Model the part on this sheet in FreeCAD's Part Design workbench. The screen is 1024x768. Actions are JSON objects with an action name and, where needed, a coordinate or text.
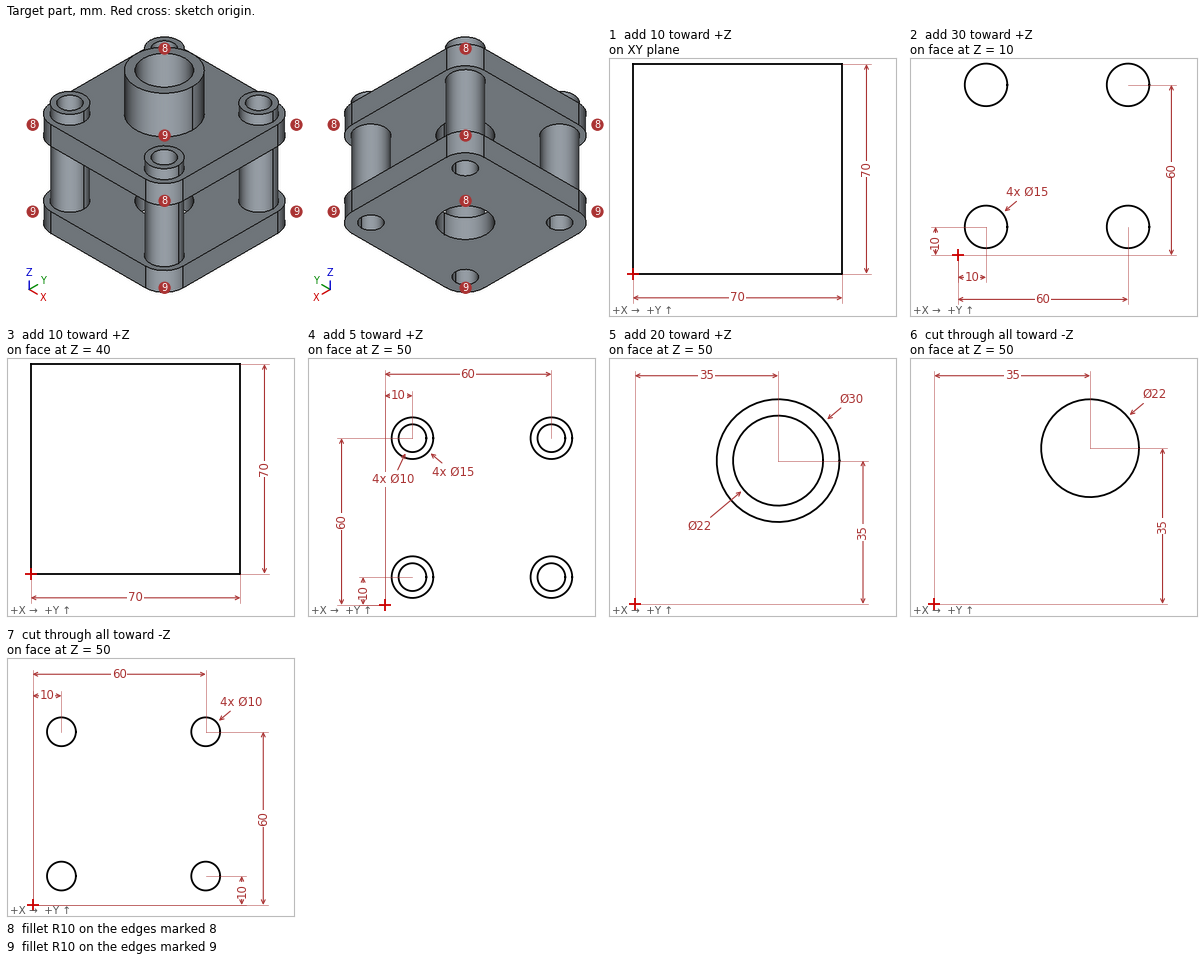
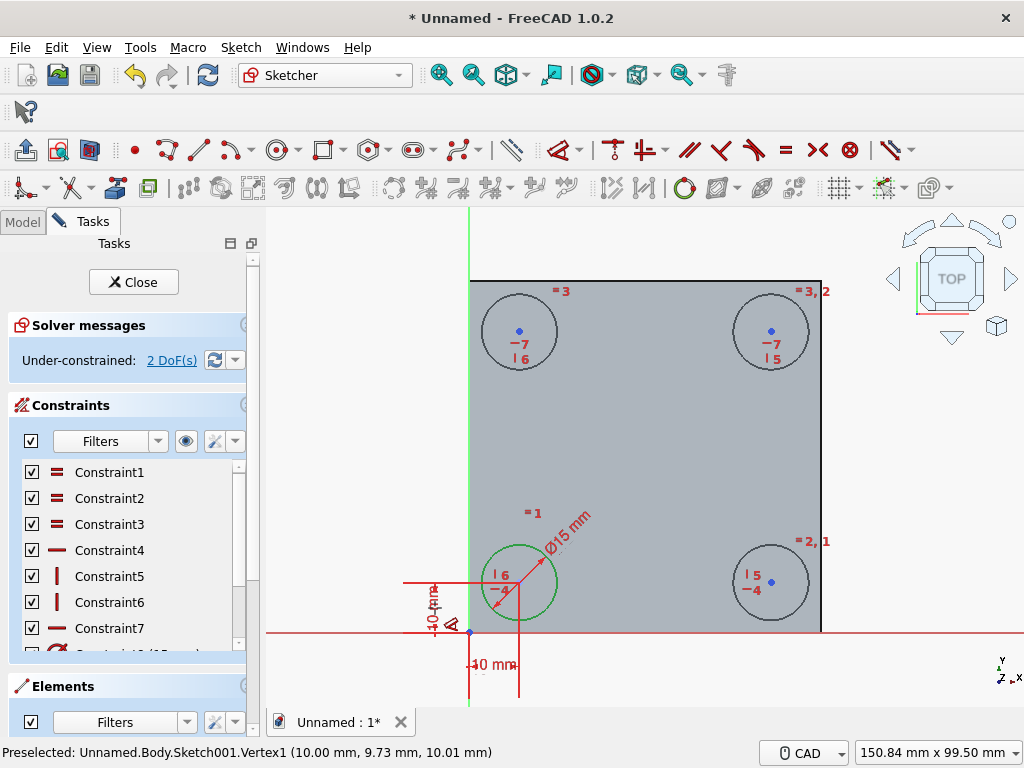
{"action": "left_click", "coordinate": [771, 583]}
{"action": "left_click", "coordinate": [620, 667]}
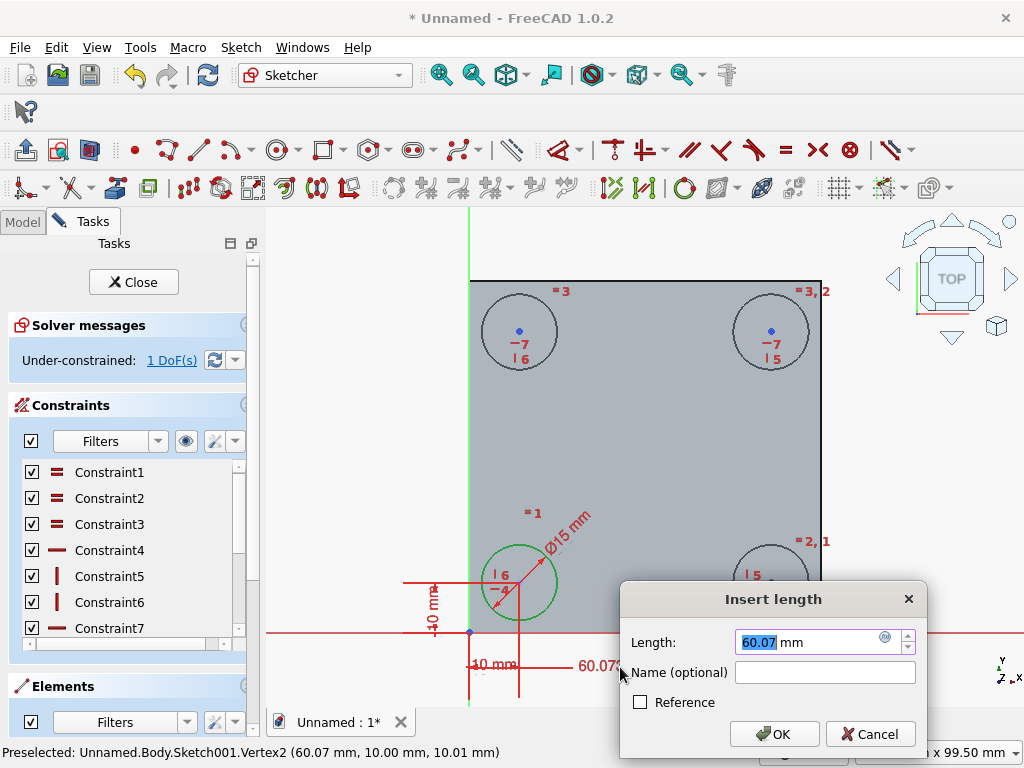
{"action": "type", "text": "60"}
{"action": "key", "text": "Return"}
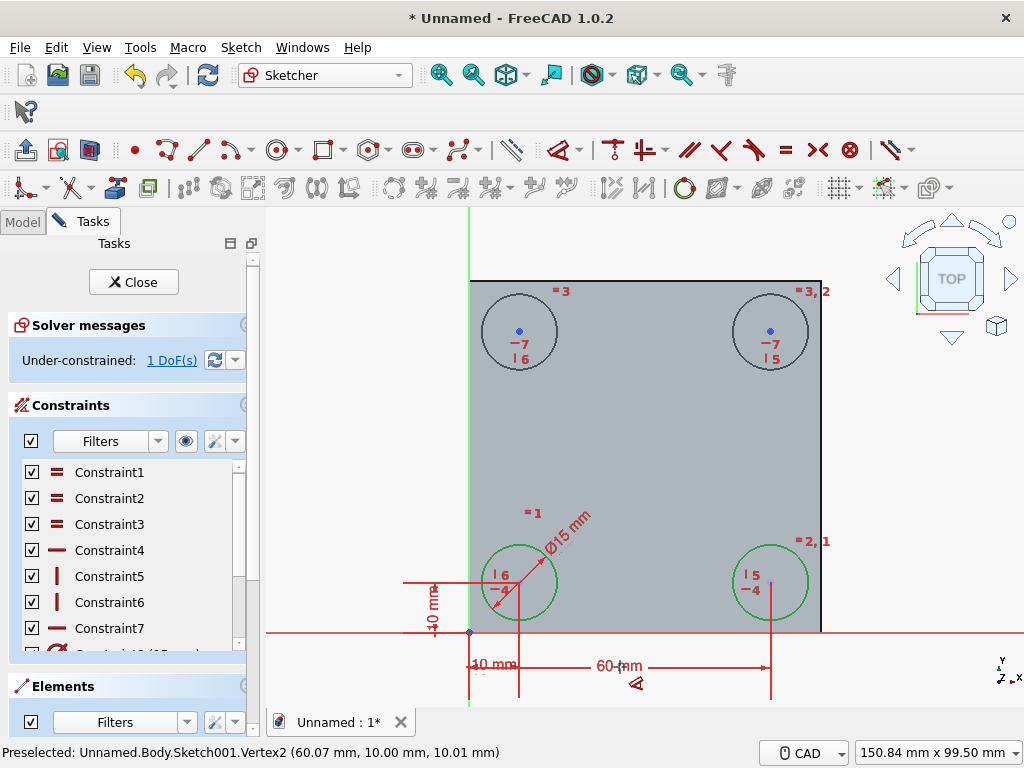
{"action": "left_click", "coordinate": [771, 332]}
{"action": "left_click", "coordinate": [435, 482]}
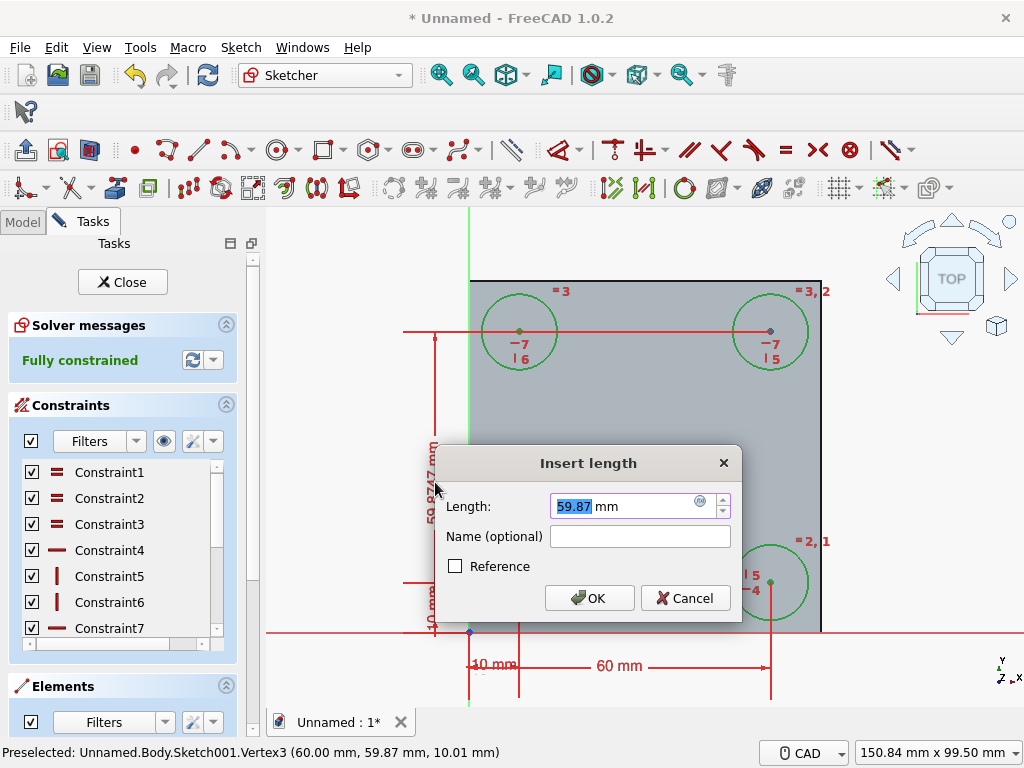
{"action": "type", "text": "60"}
{"action": "key", "text": "Return"}
{"action": "key", "text": "Escape"}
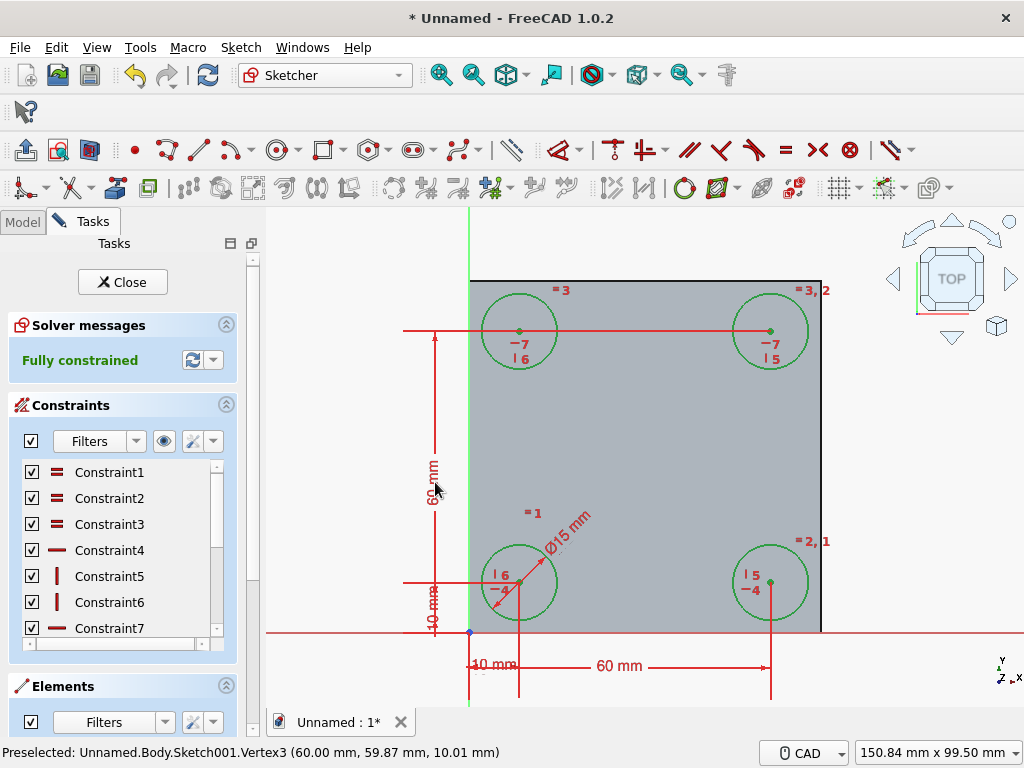
{"action": "left_click", "coordinate": [123, 282]}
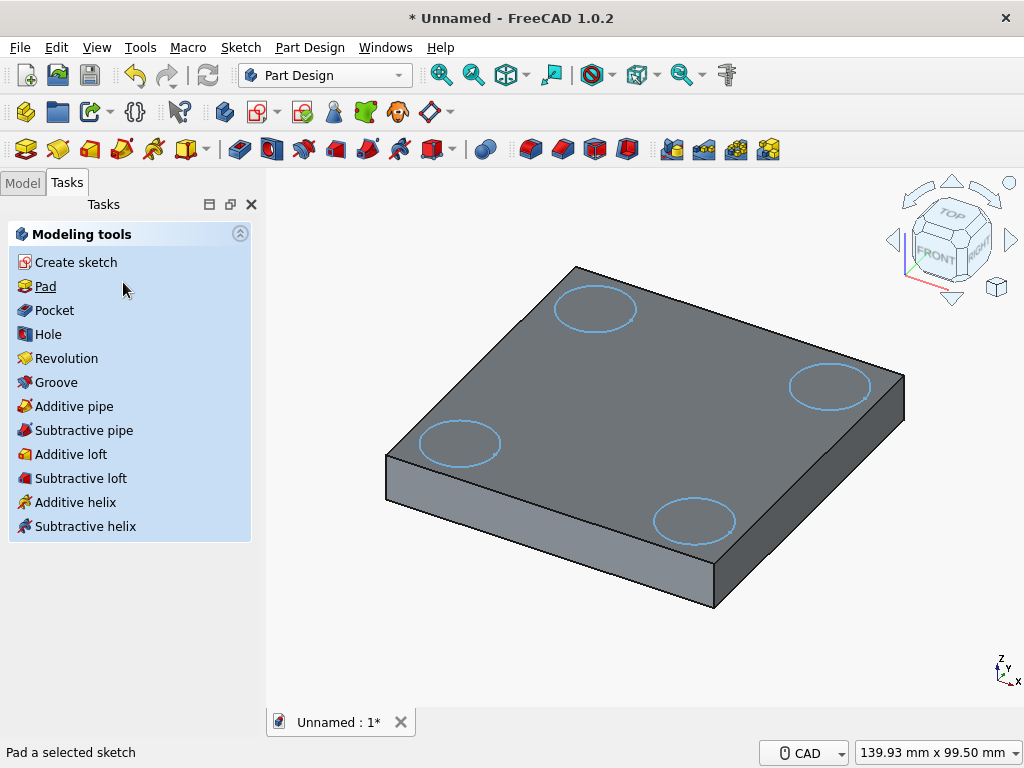
{"action": "left_click", "coordinate": [26, 150]}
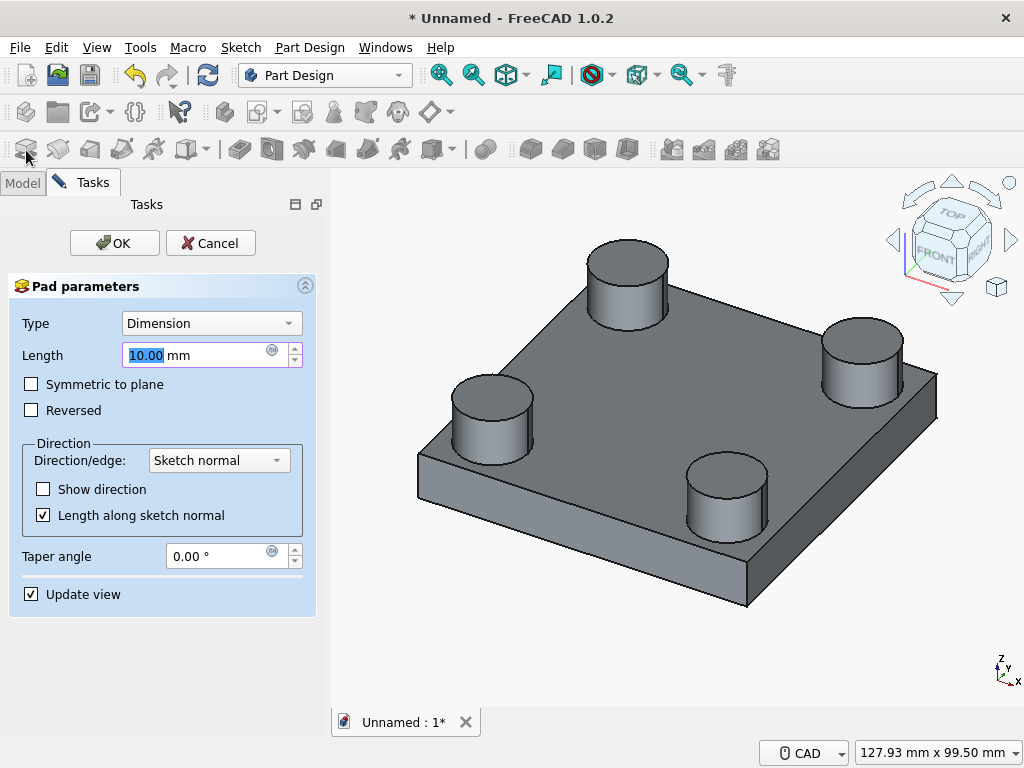
{"action": "type", "text": "30"}
{"action": "key", "text": "Tab"}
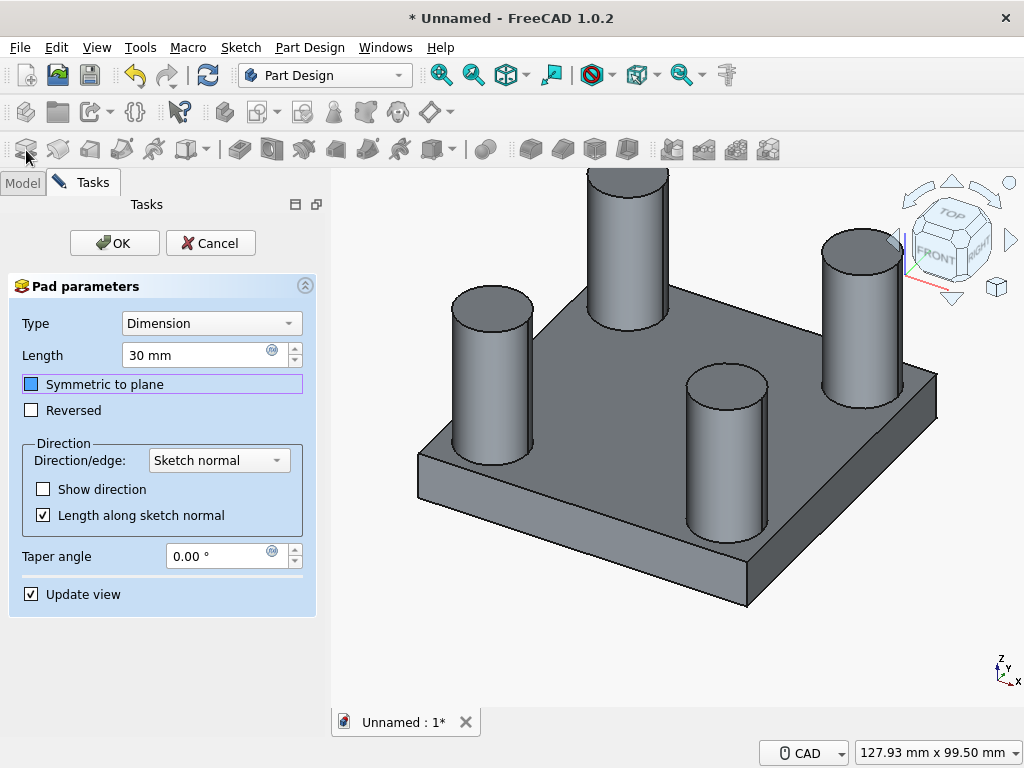
{"action": "left_click", "coordinate": [115, 243]}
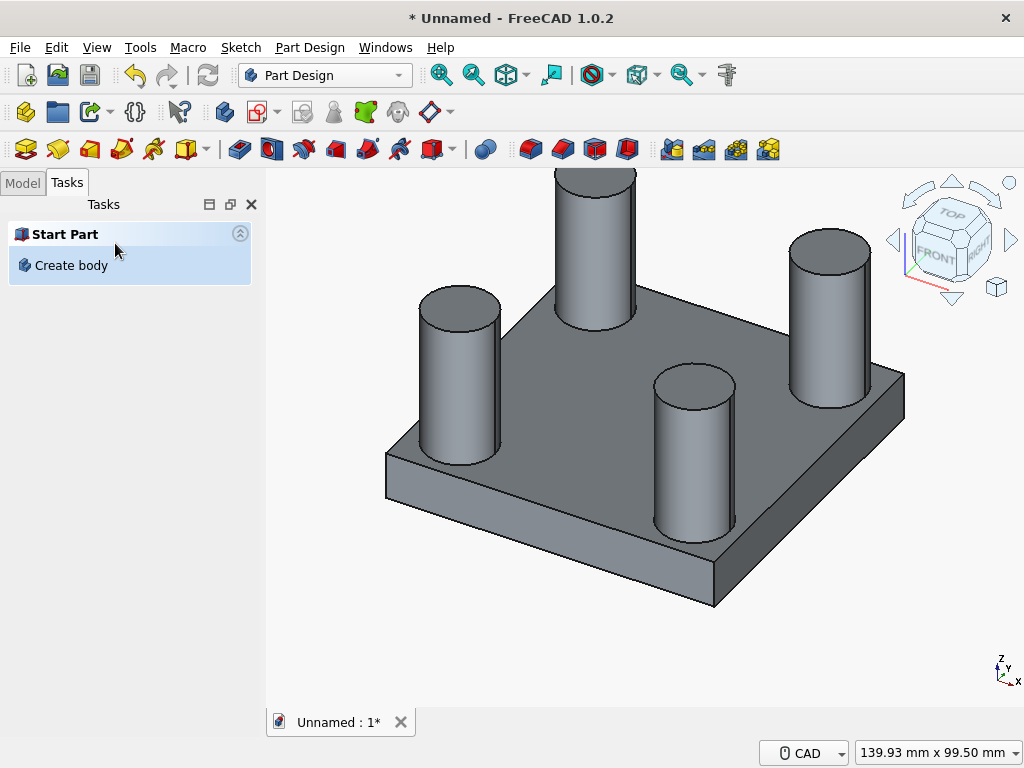
{"action": "key", "text": "v f"}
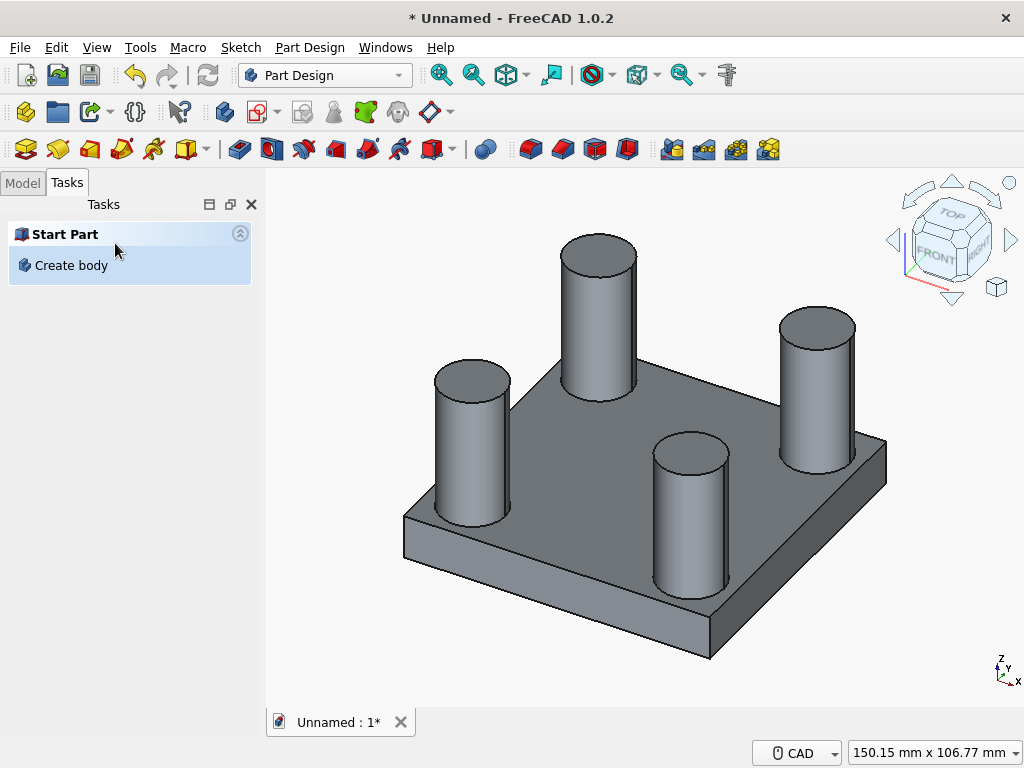
{"action": "left_click", "coordinate": [817, 327]}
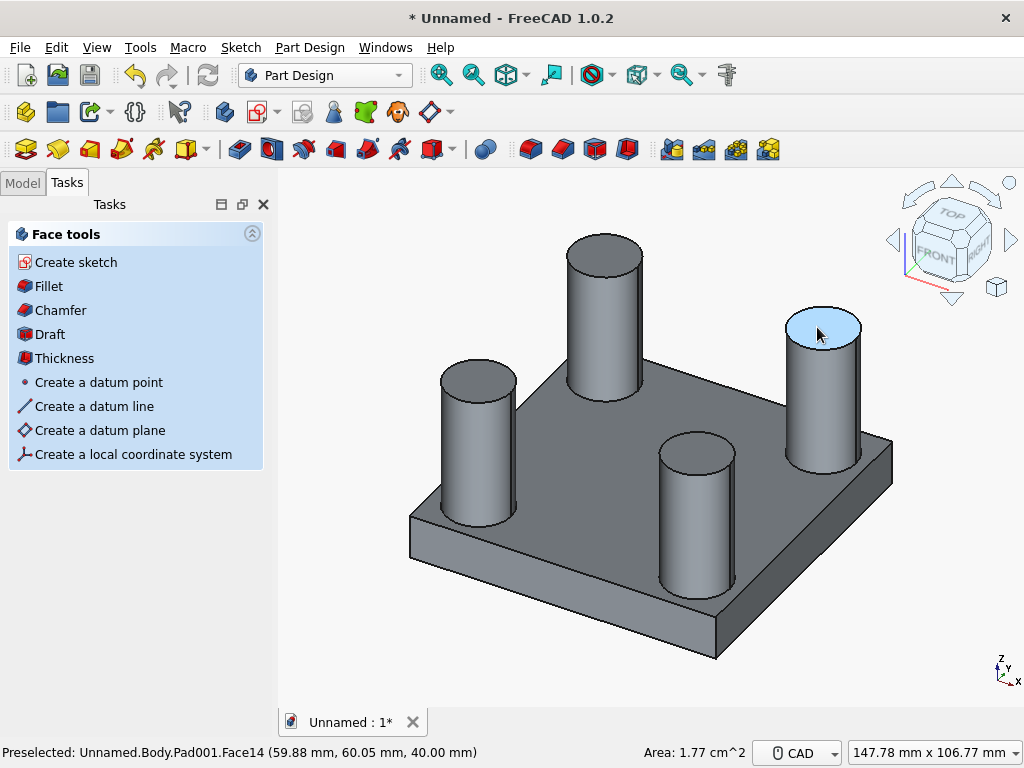
{"action": "left_click", "coordinate": [258, 112]}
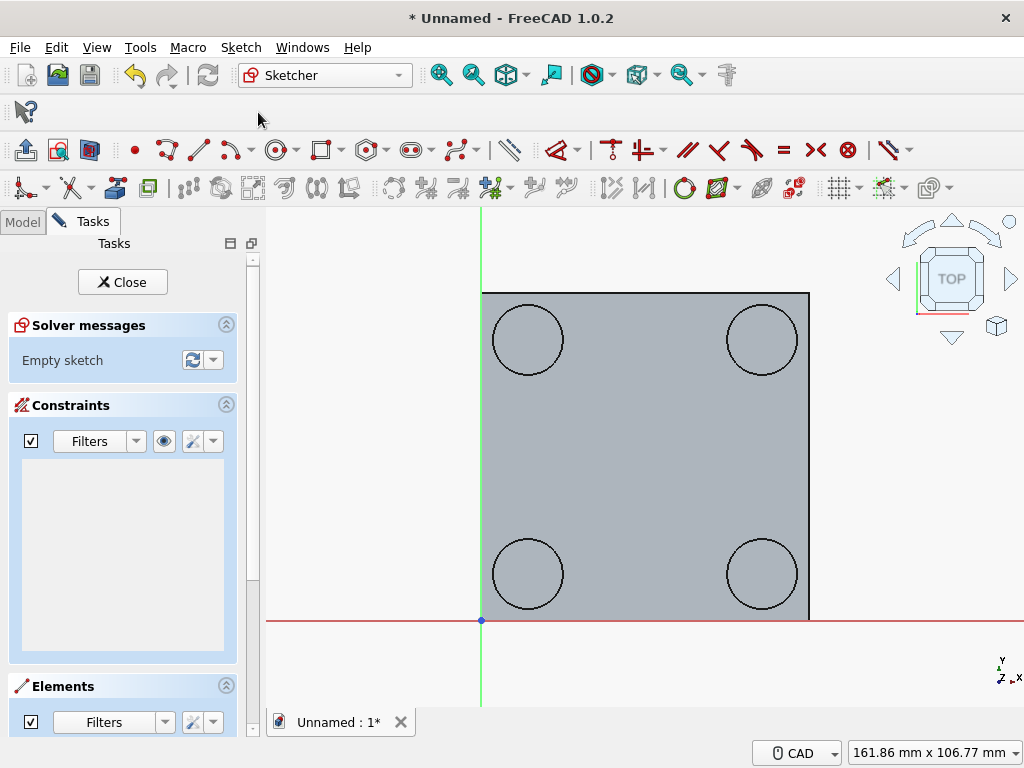
{"action": "left_click", "coordinate": [322, 150]}